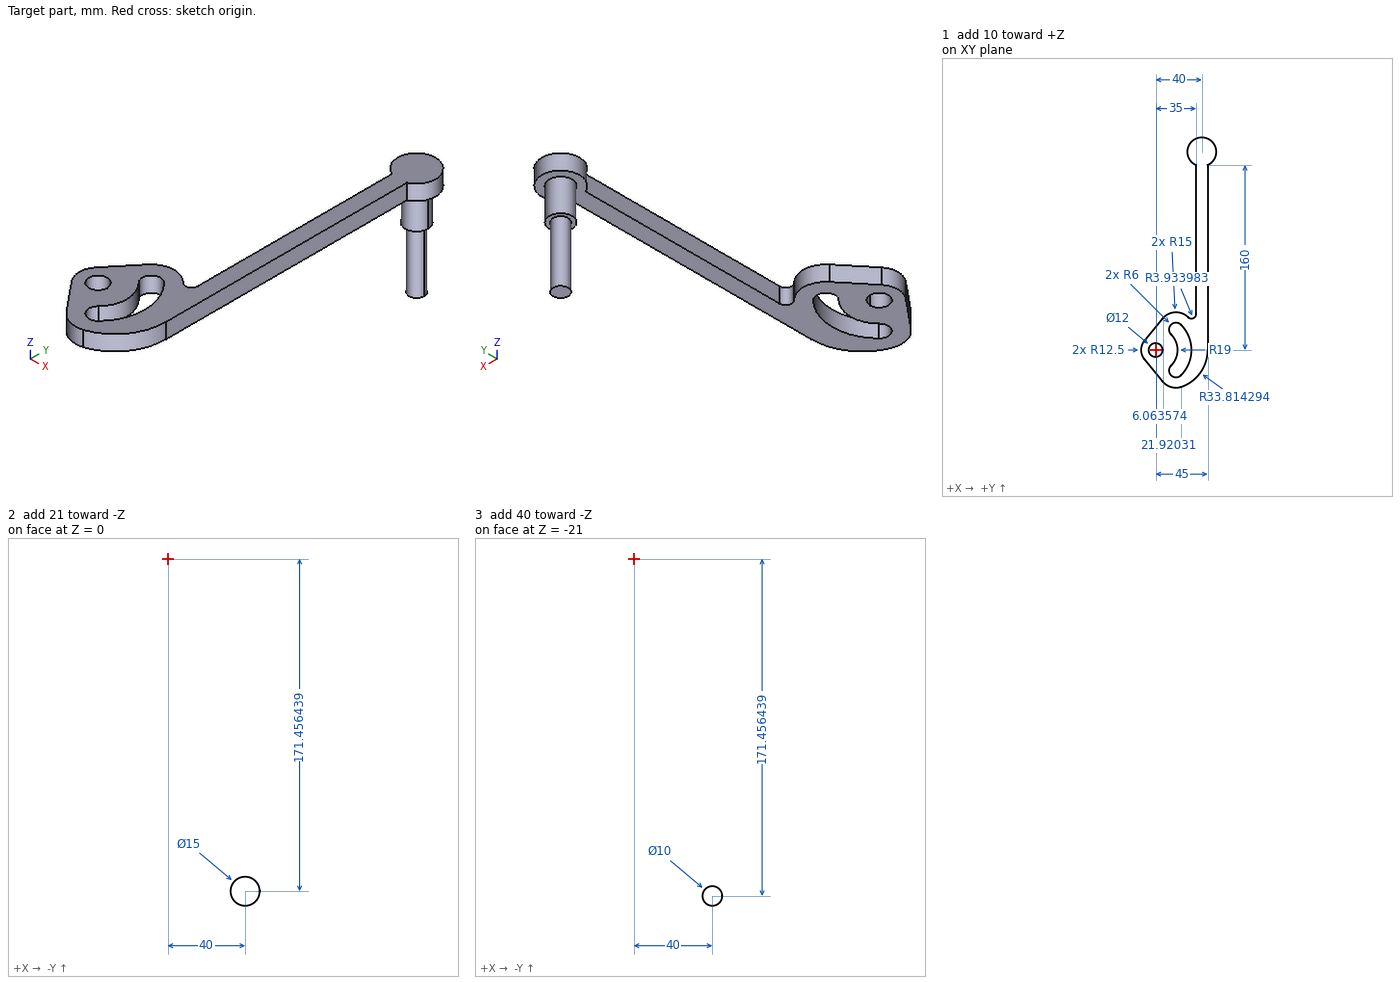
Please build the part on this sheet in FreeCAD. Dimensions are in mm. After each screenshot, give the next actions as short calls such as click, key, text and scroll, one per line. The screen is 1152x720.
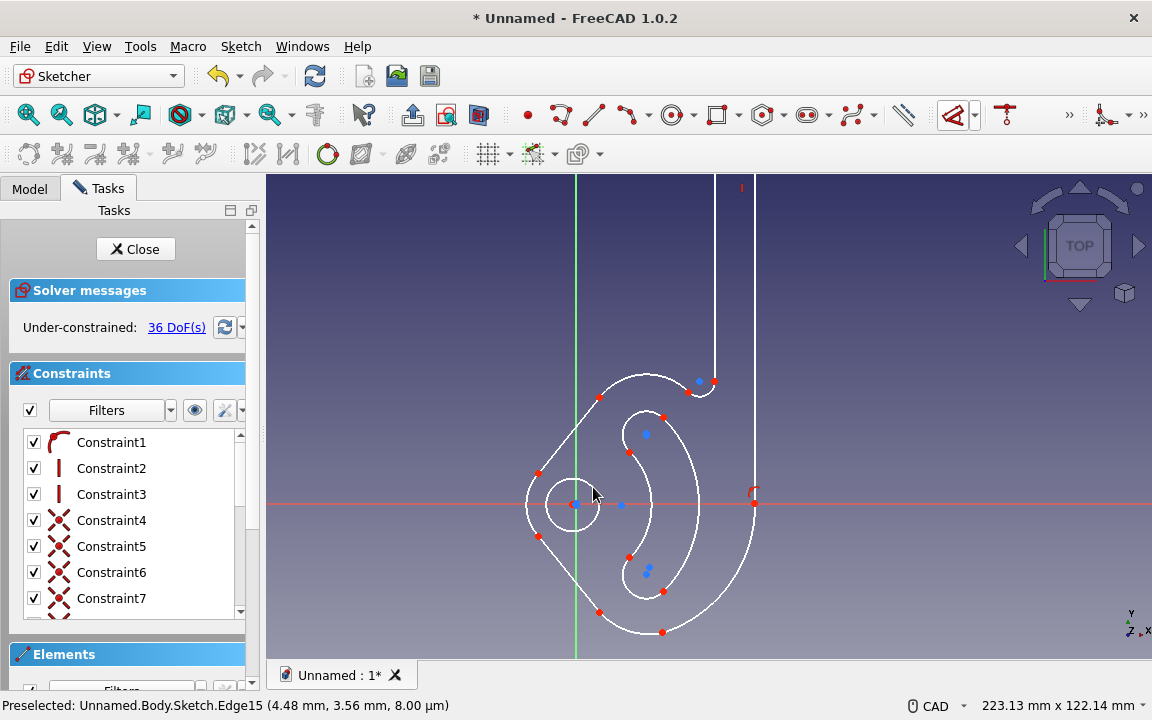
click(557, 451)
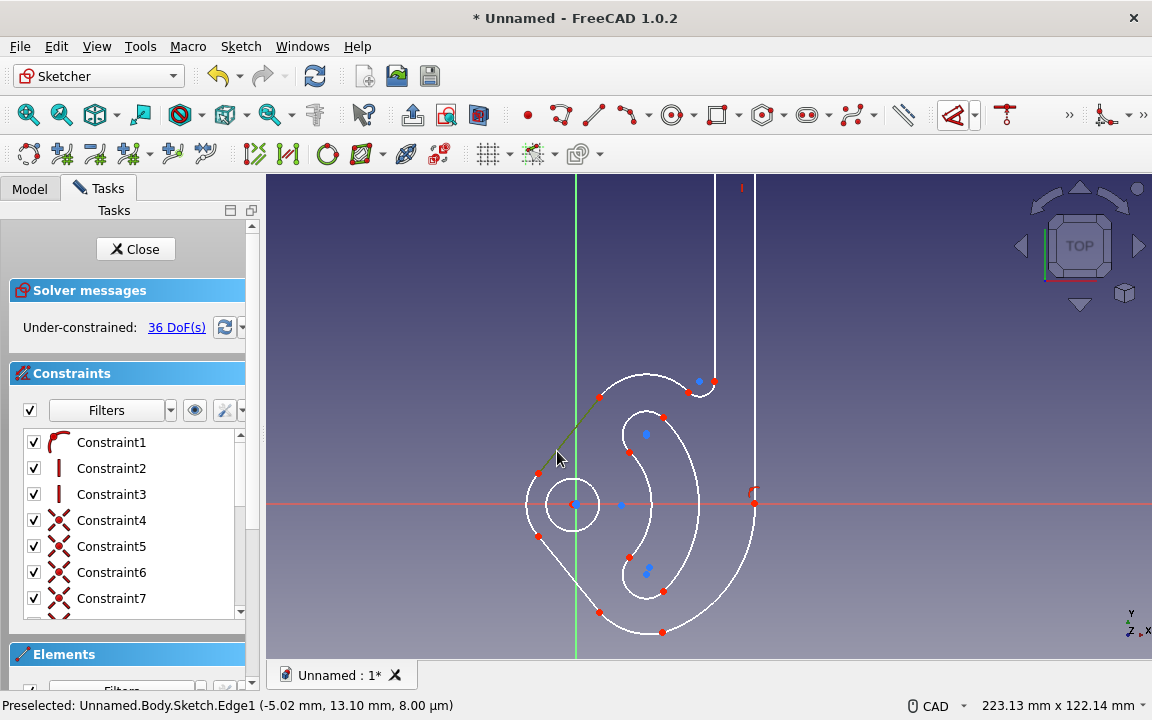
click(528, 491)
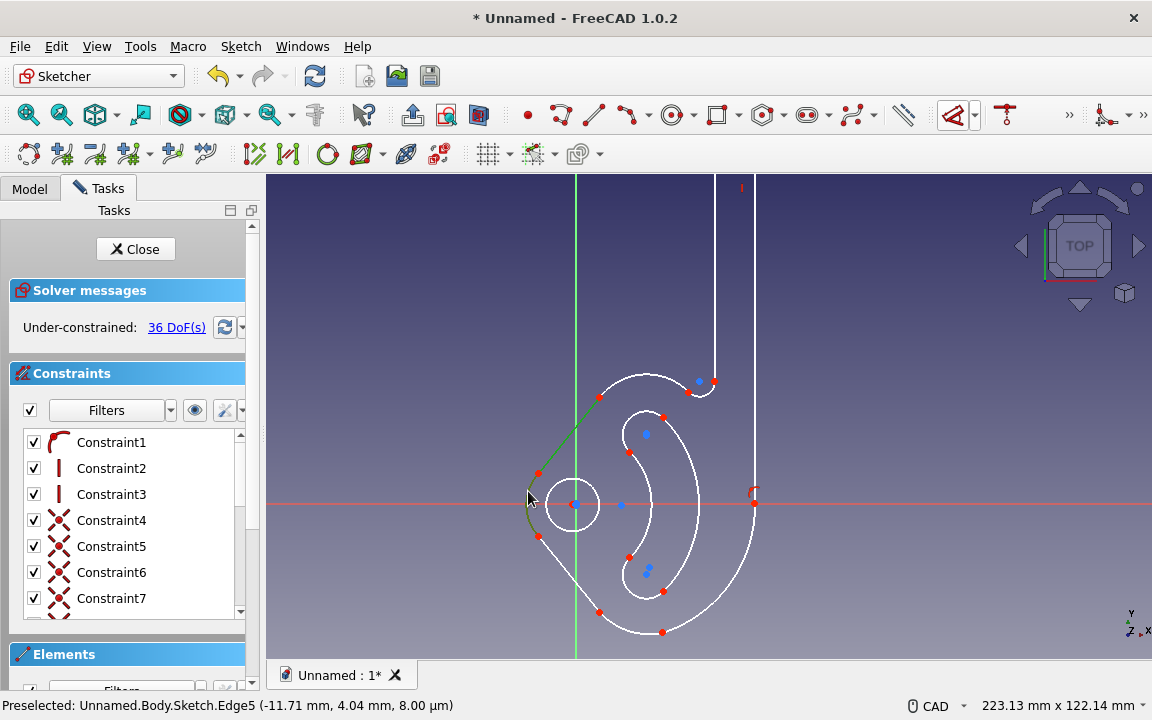
key(t)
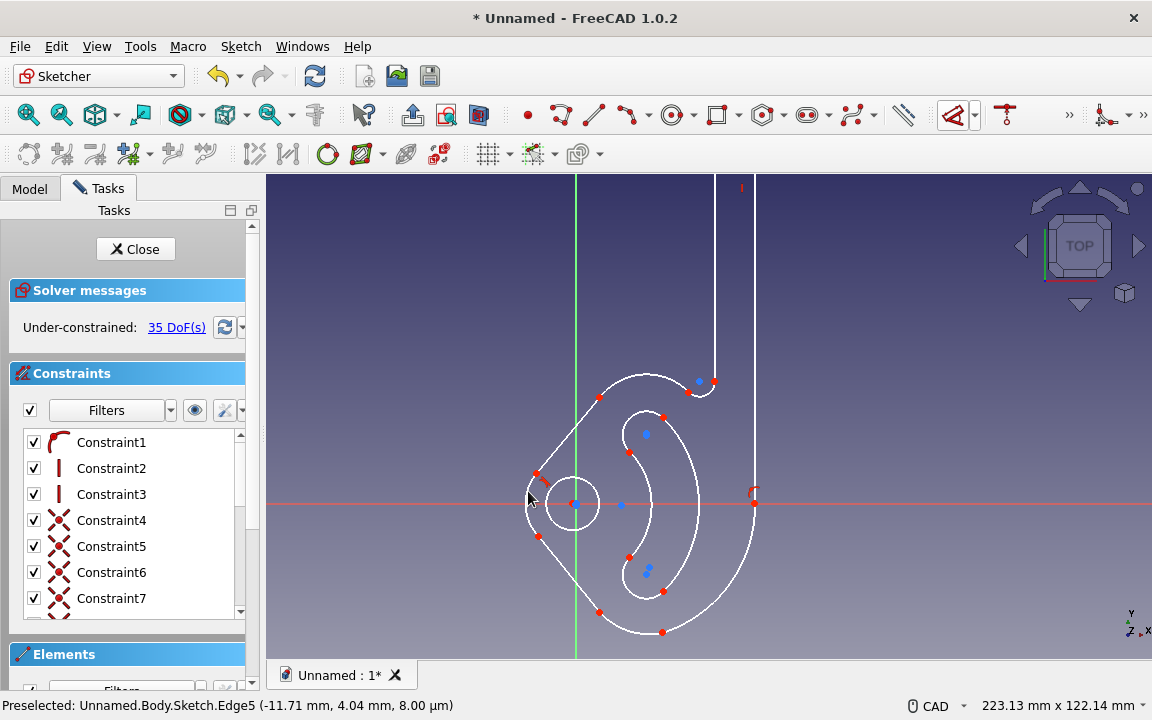
click(555, 451)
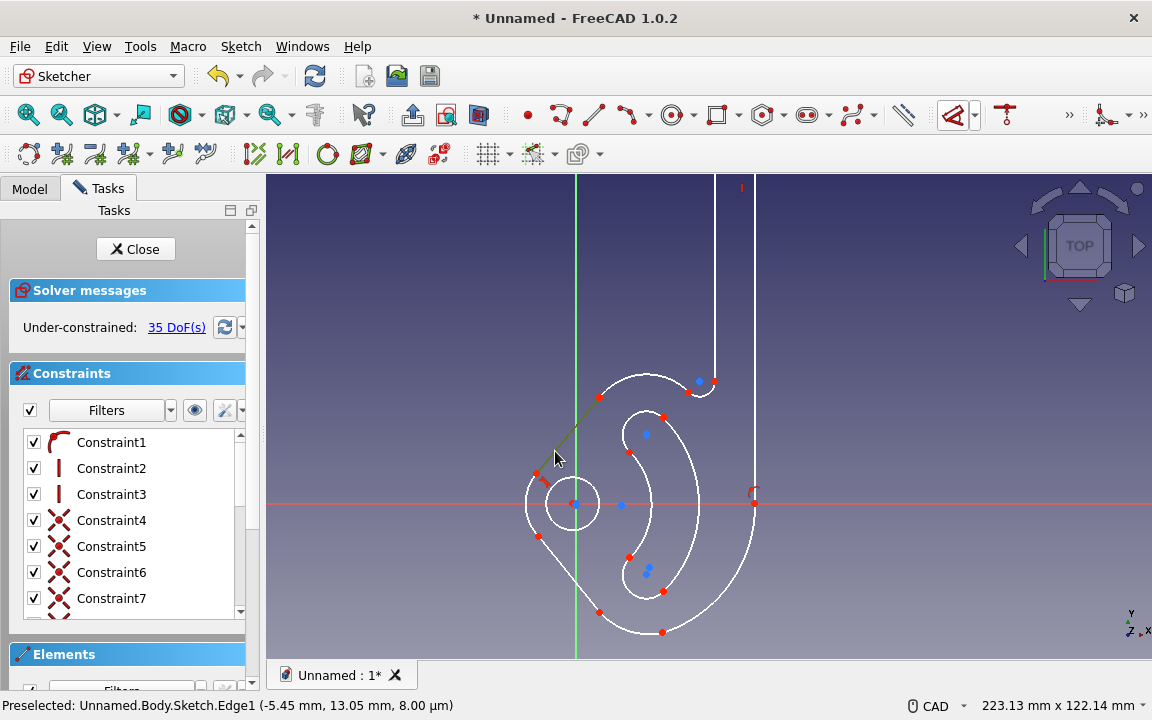
click(663, 377)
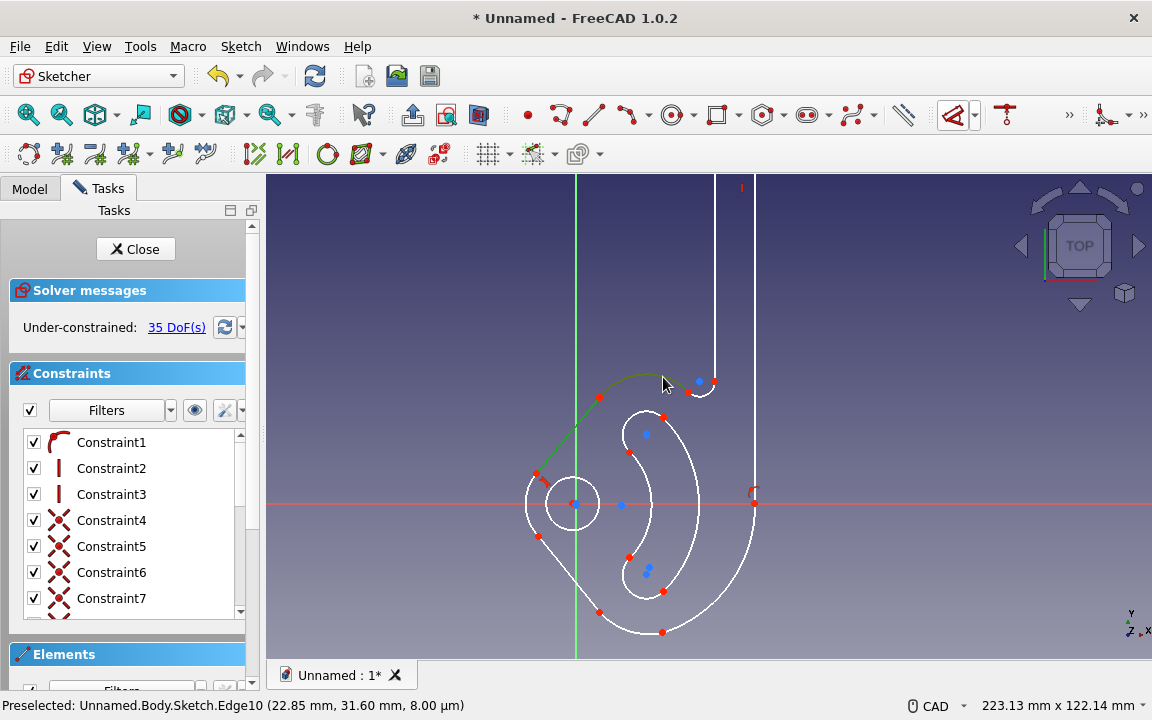
key(t)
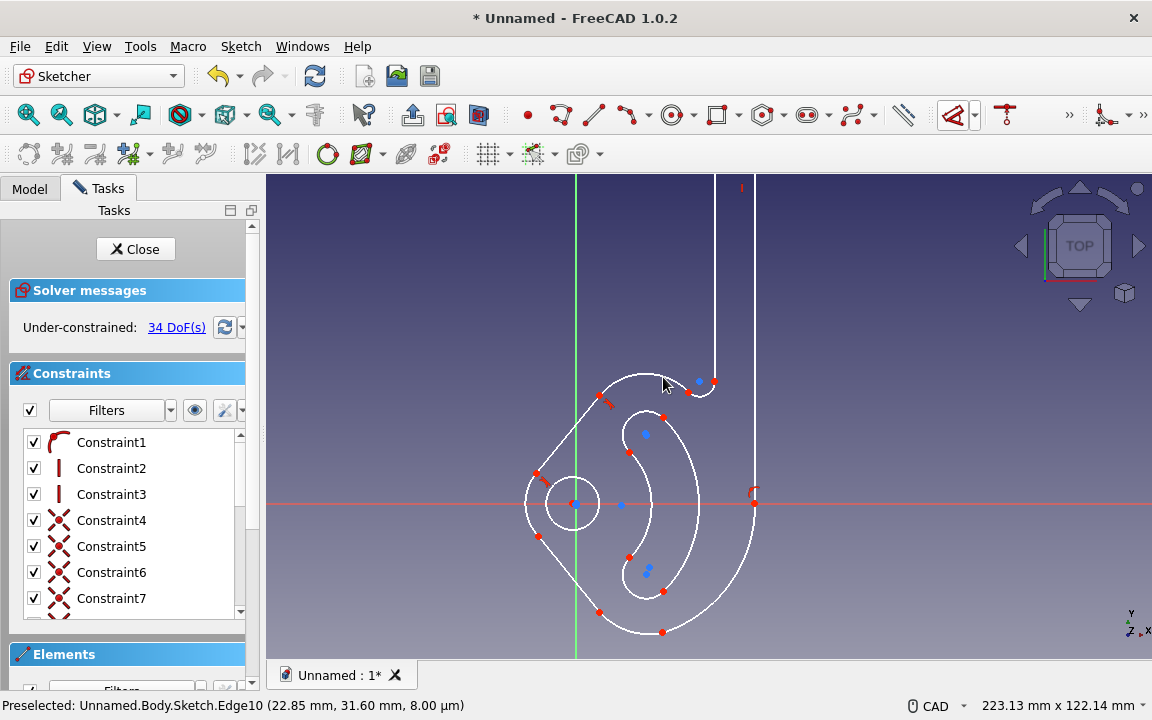
click(557, 559)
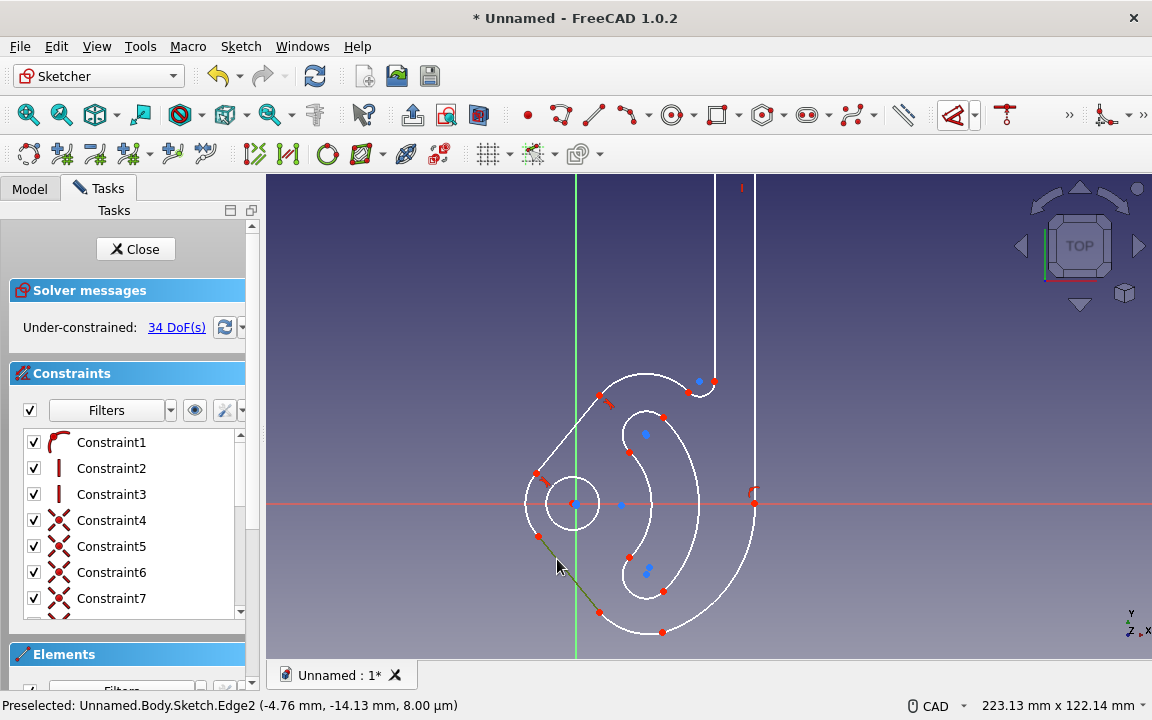
click(527, 492)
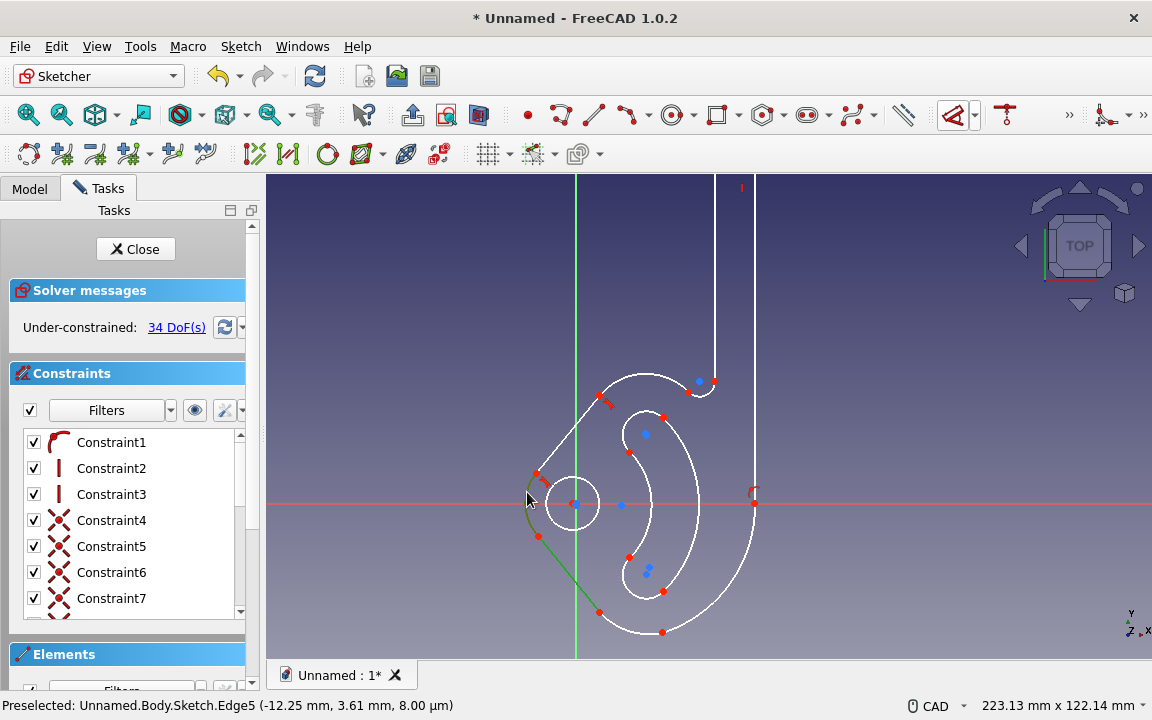
key(t)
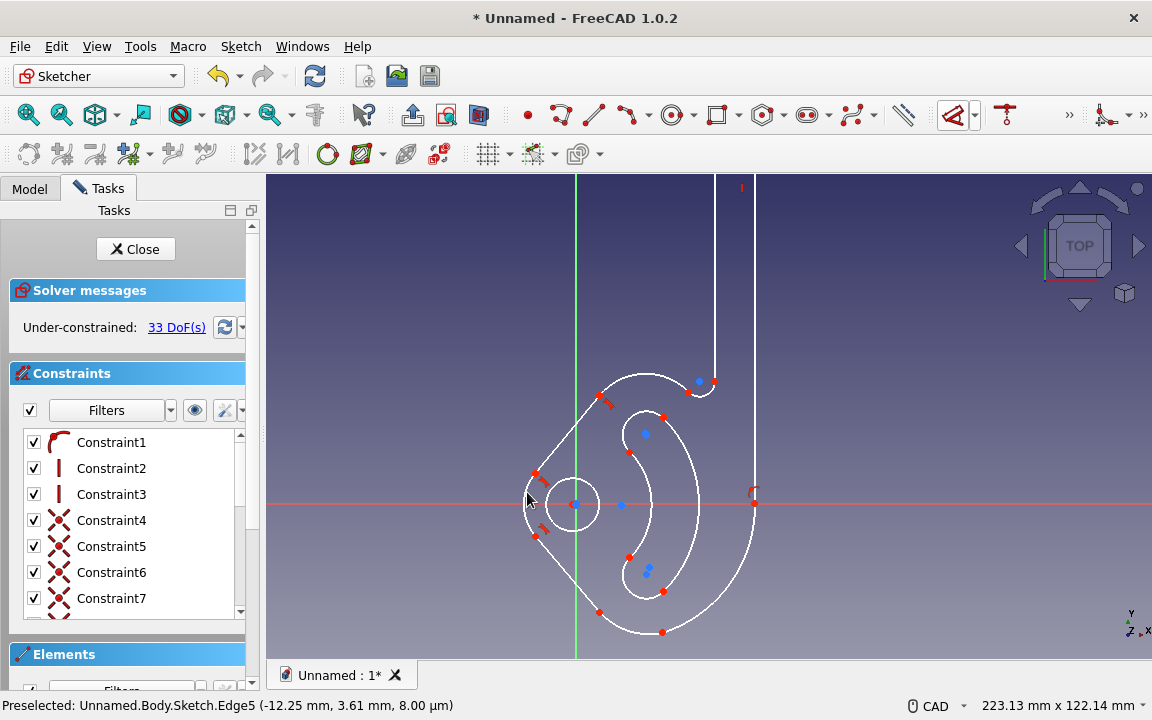
click(555, 559)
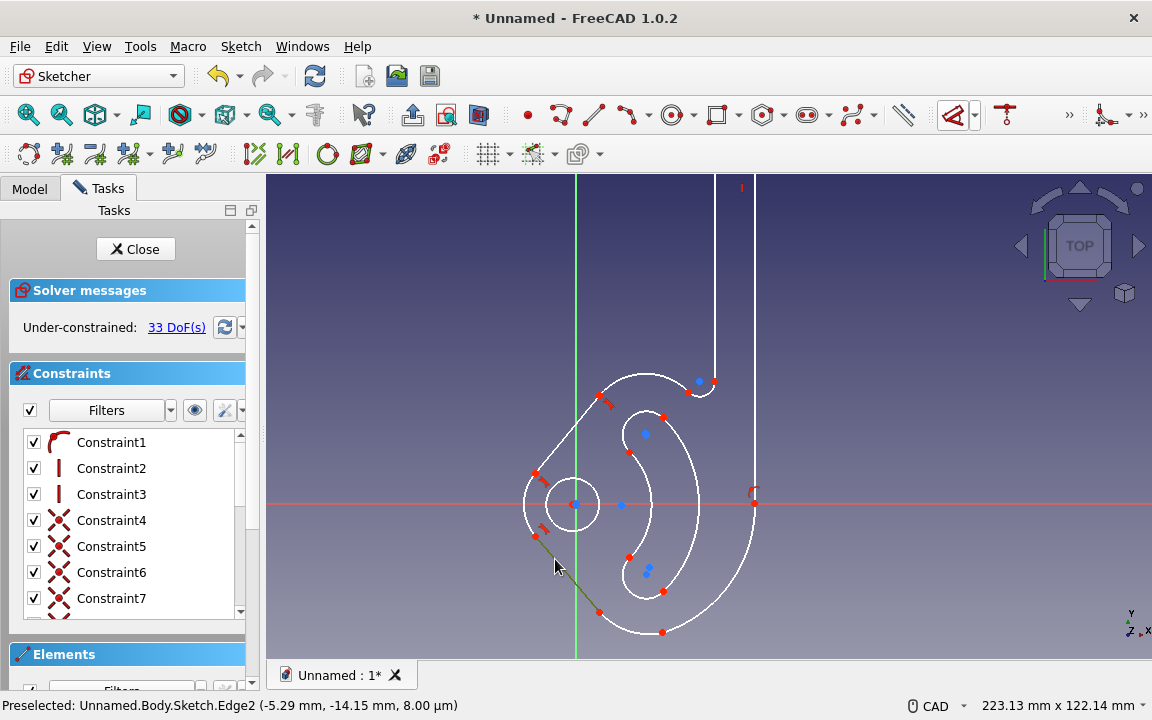
click(616, 625)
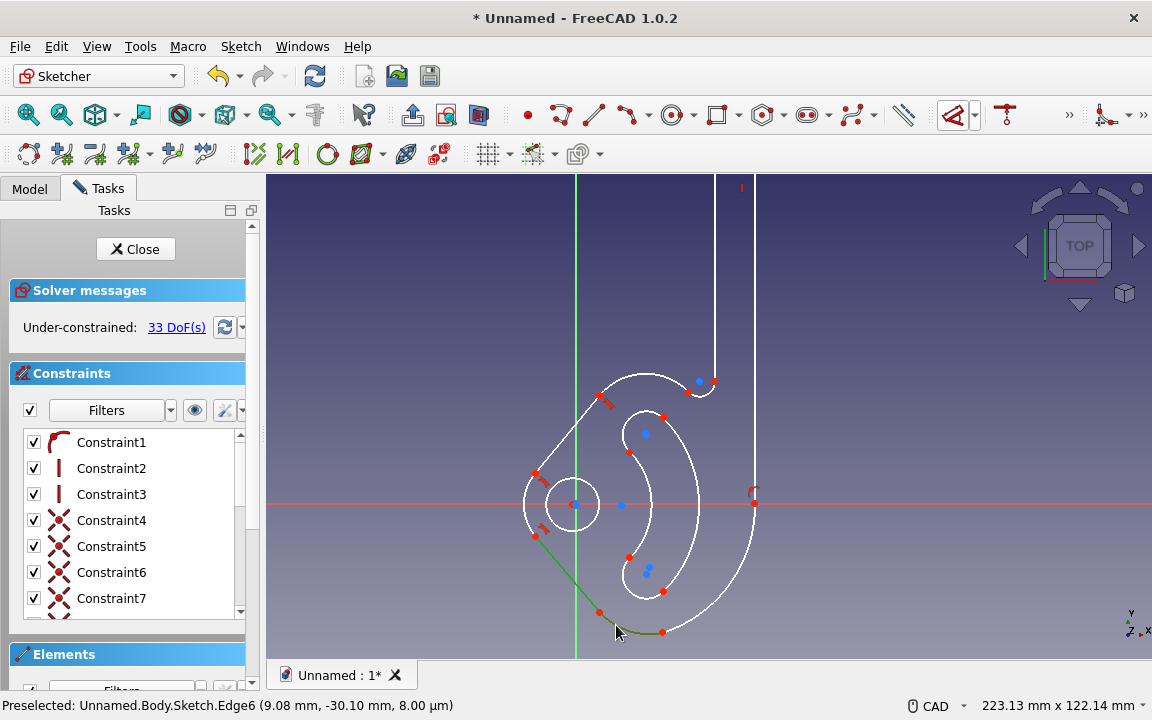
key(t)